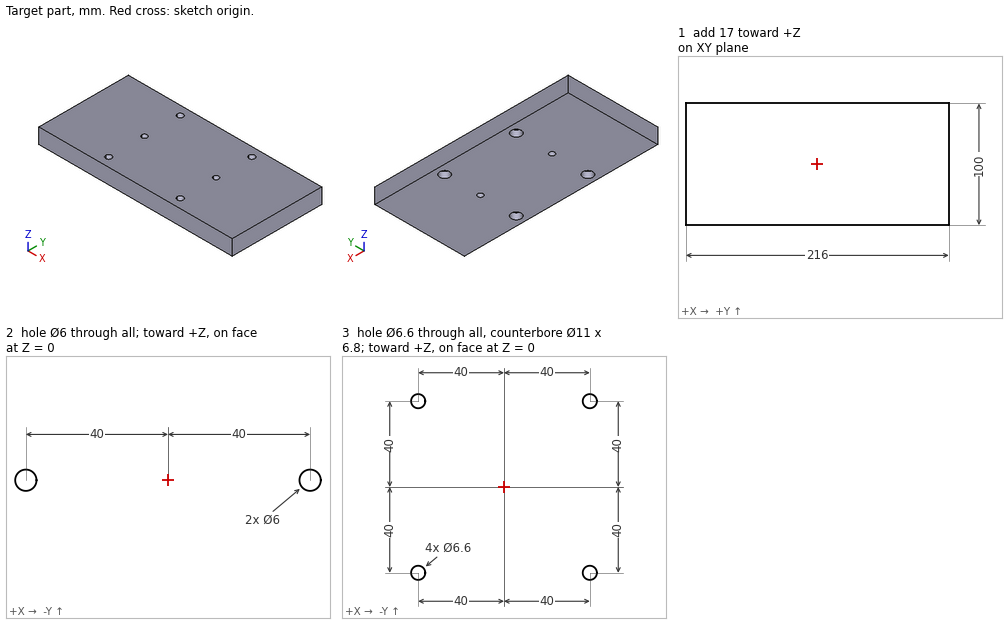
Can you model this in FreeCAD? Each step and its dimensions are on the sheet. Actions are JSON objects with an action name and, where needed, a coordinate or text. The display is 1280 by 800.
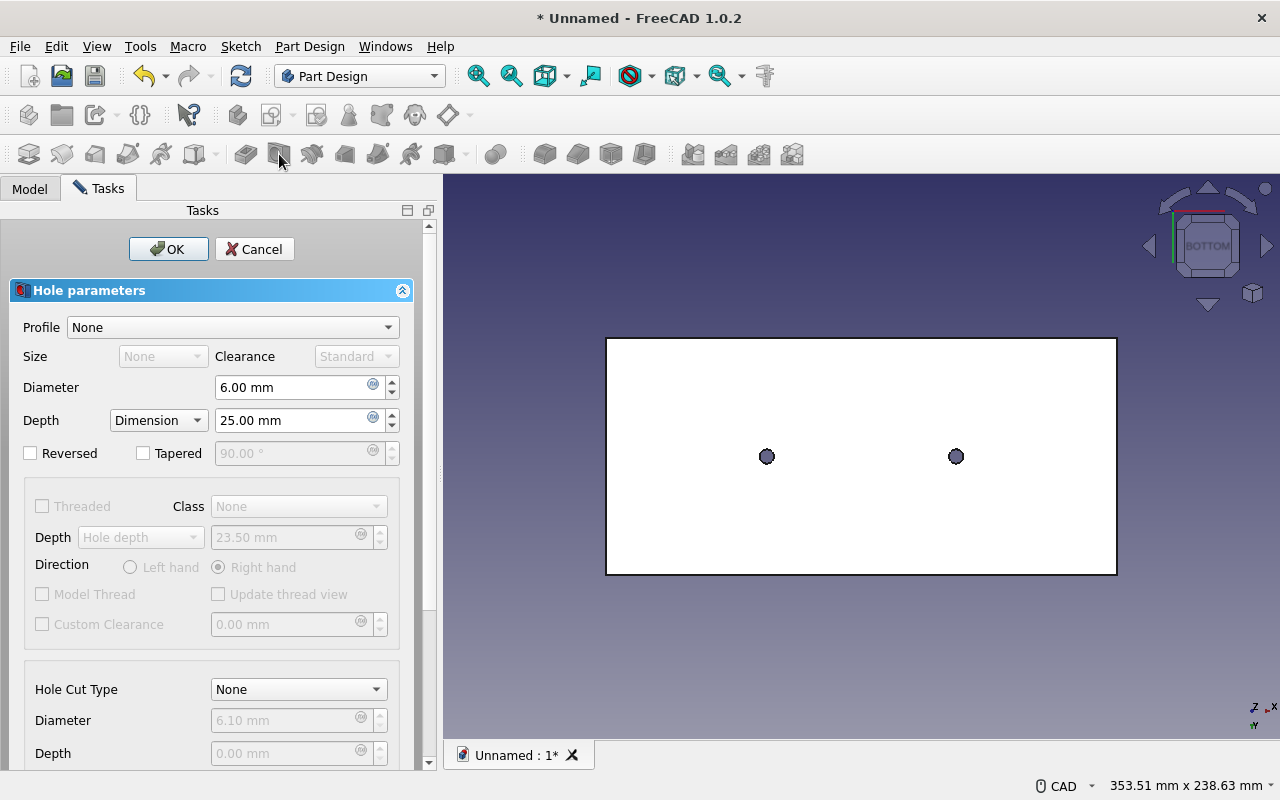
{"action": "triple_click", "coordinate": [300, 388]}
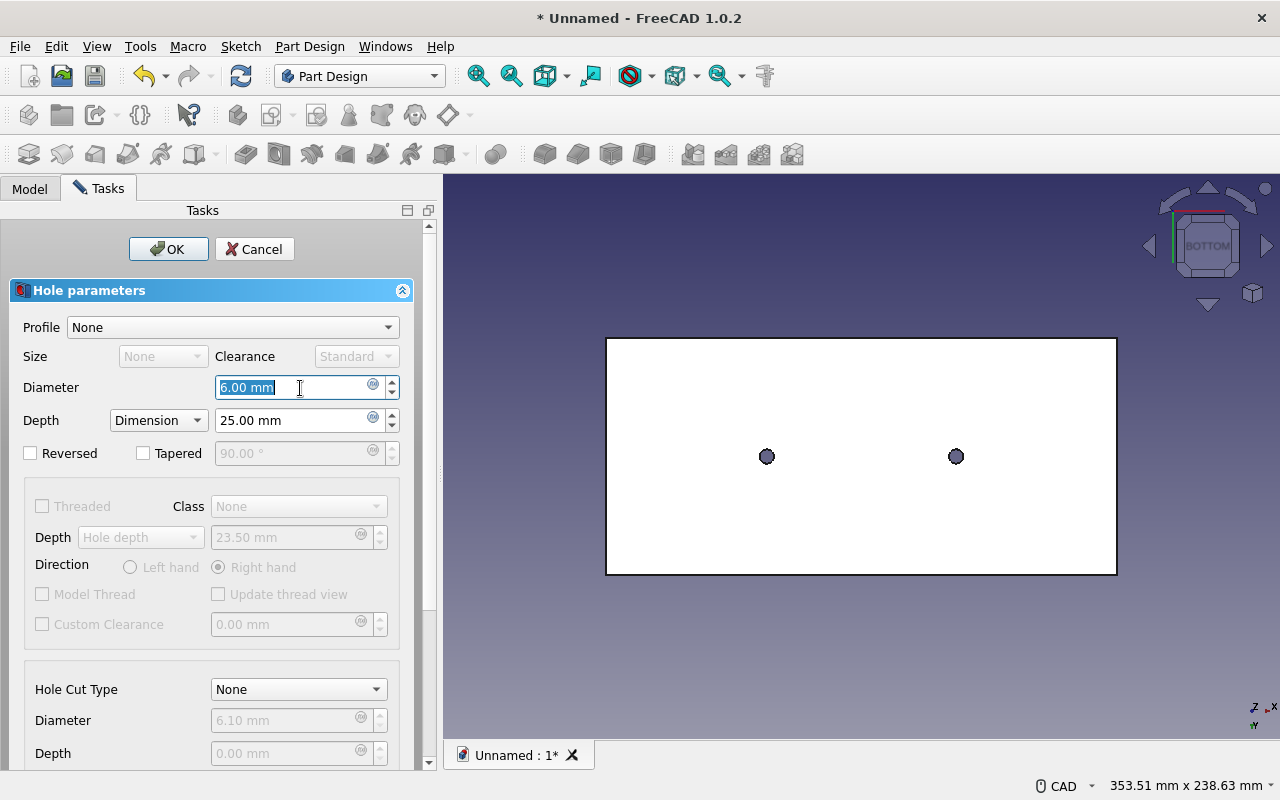
{"action": "type", "text": "6"}
{"action": "key", "text": "Tab"}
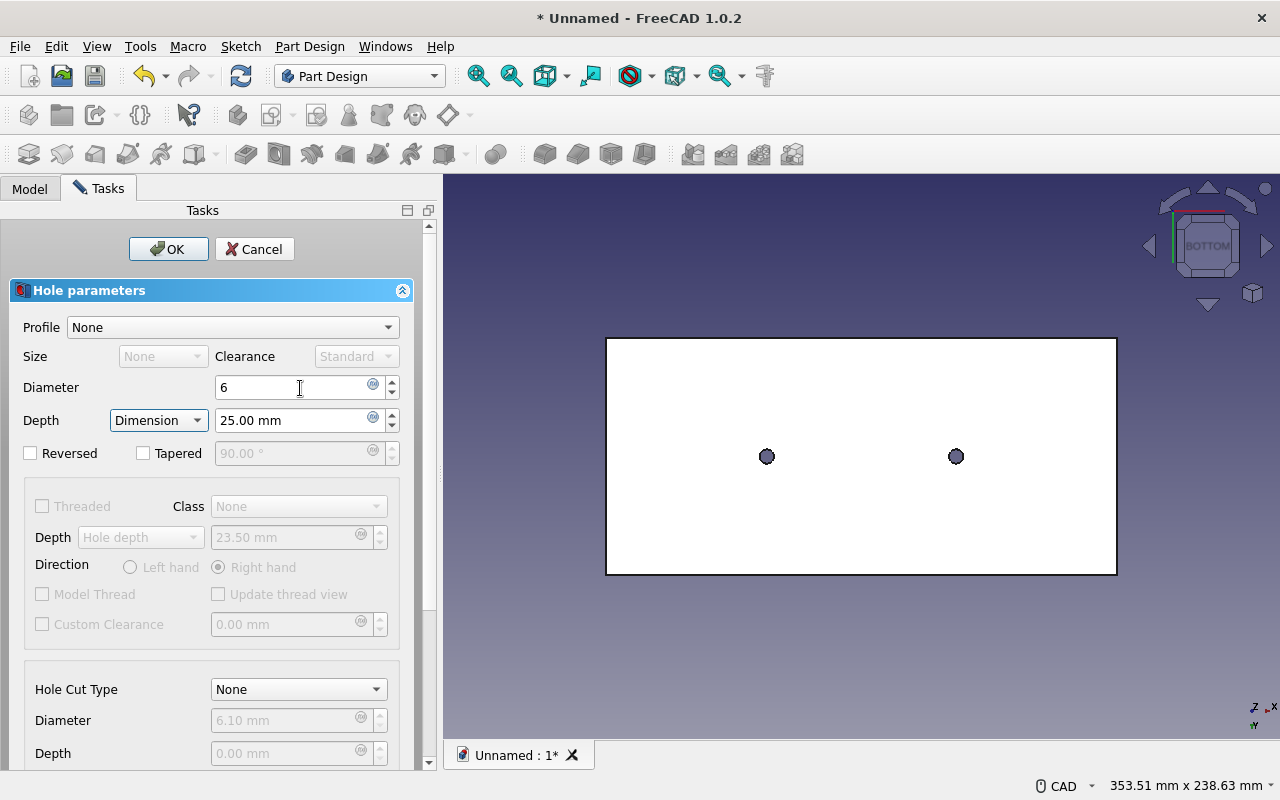
{"action": "left_click", "coordinate": [160, 420]}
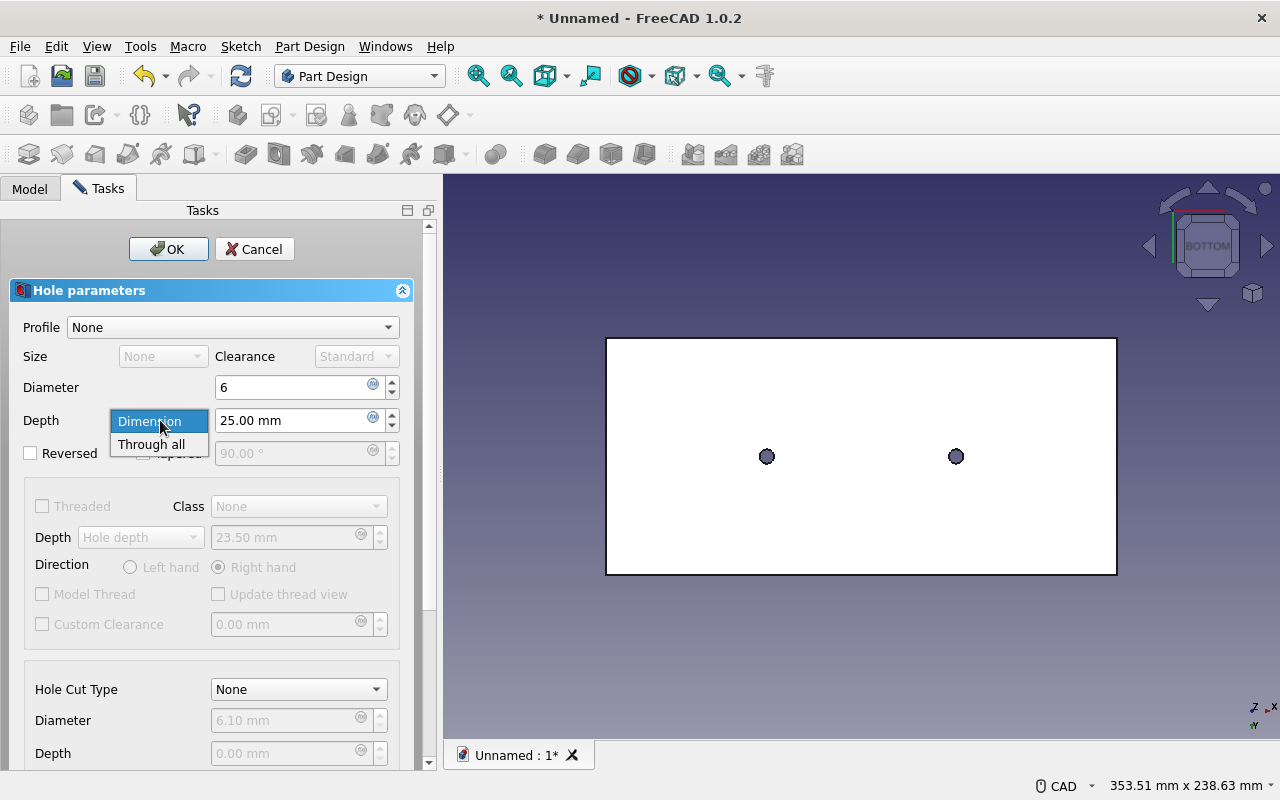
{"action": "left_click", "coordinate": [158, 444]}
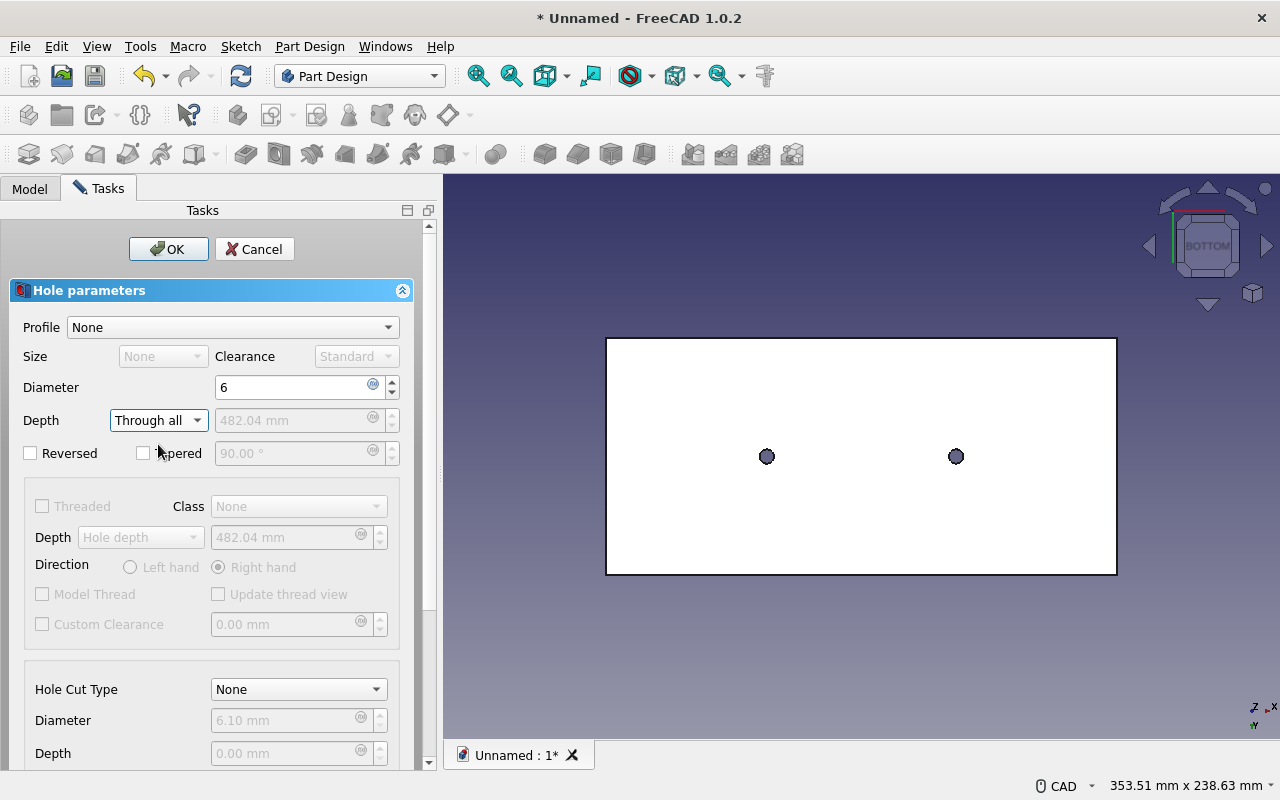
{"action": "left_click", "coordinate": [169, 249]}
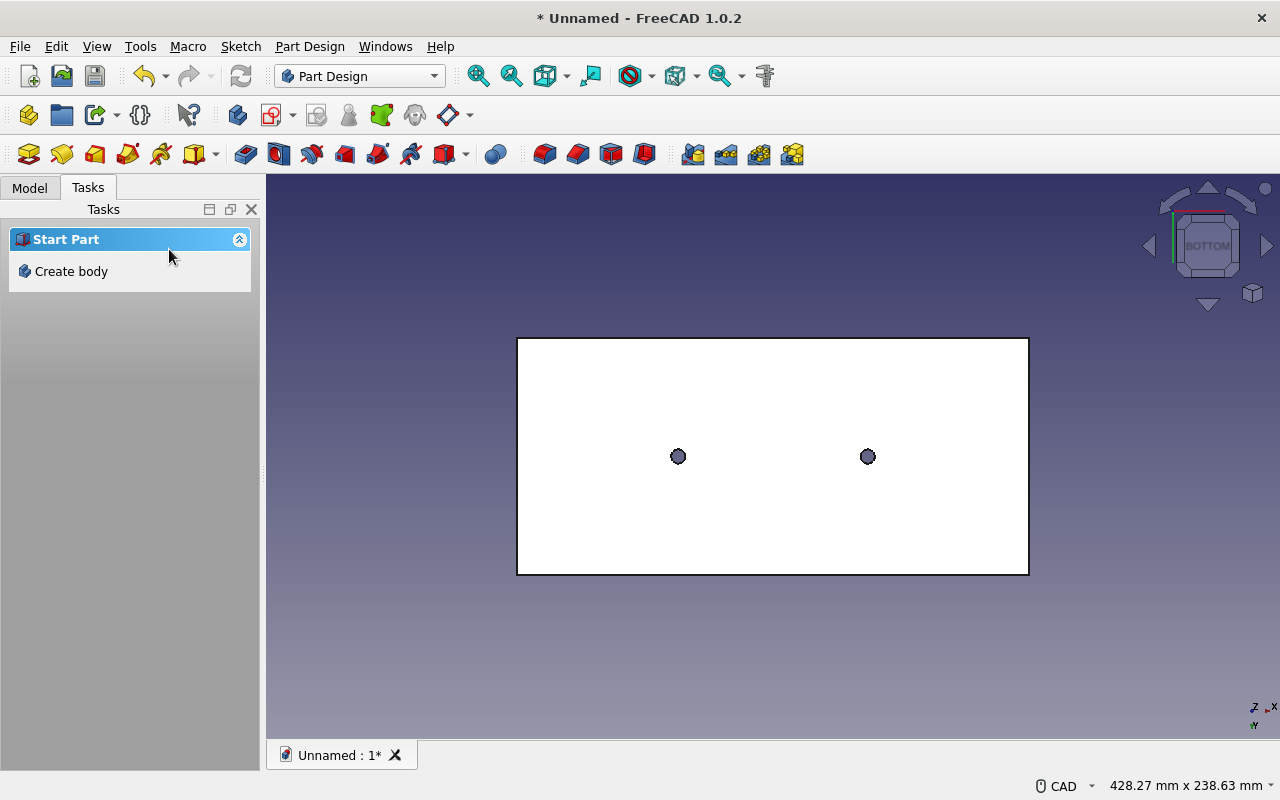
{"action": "left_click", "coordinate": [773, 456]}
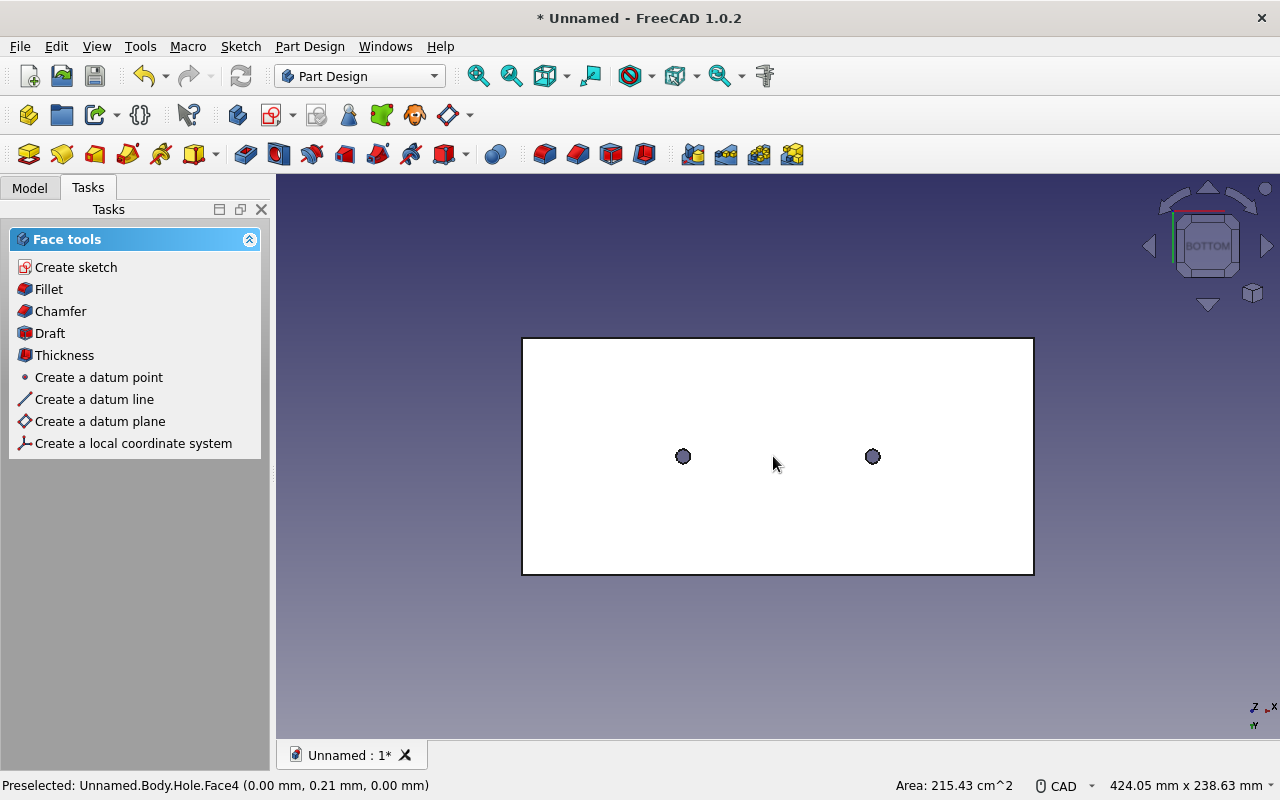
{"action": "left_click", "coordinate": [270, 116]}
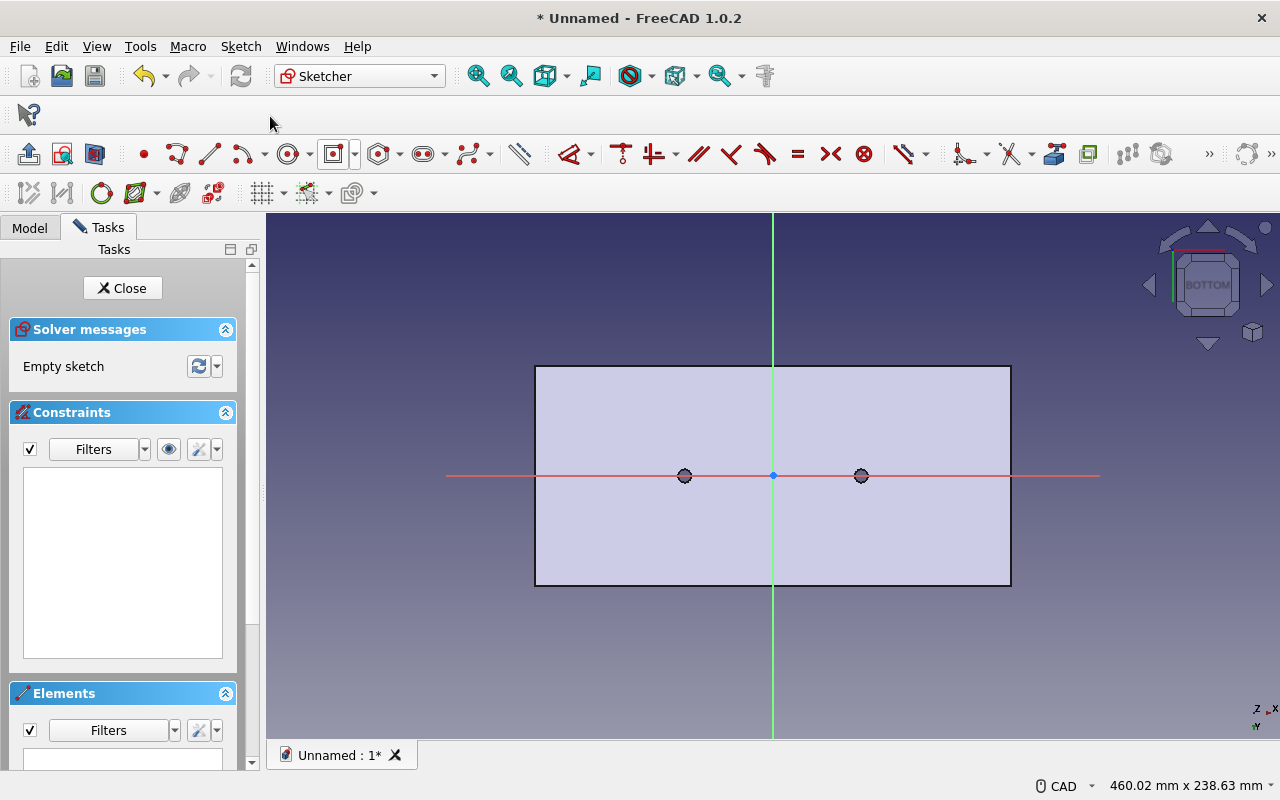
{"action": "scroll", "coordinate": [856, 476], "scroll_direction": "up", "scroll_amount": 3}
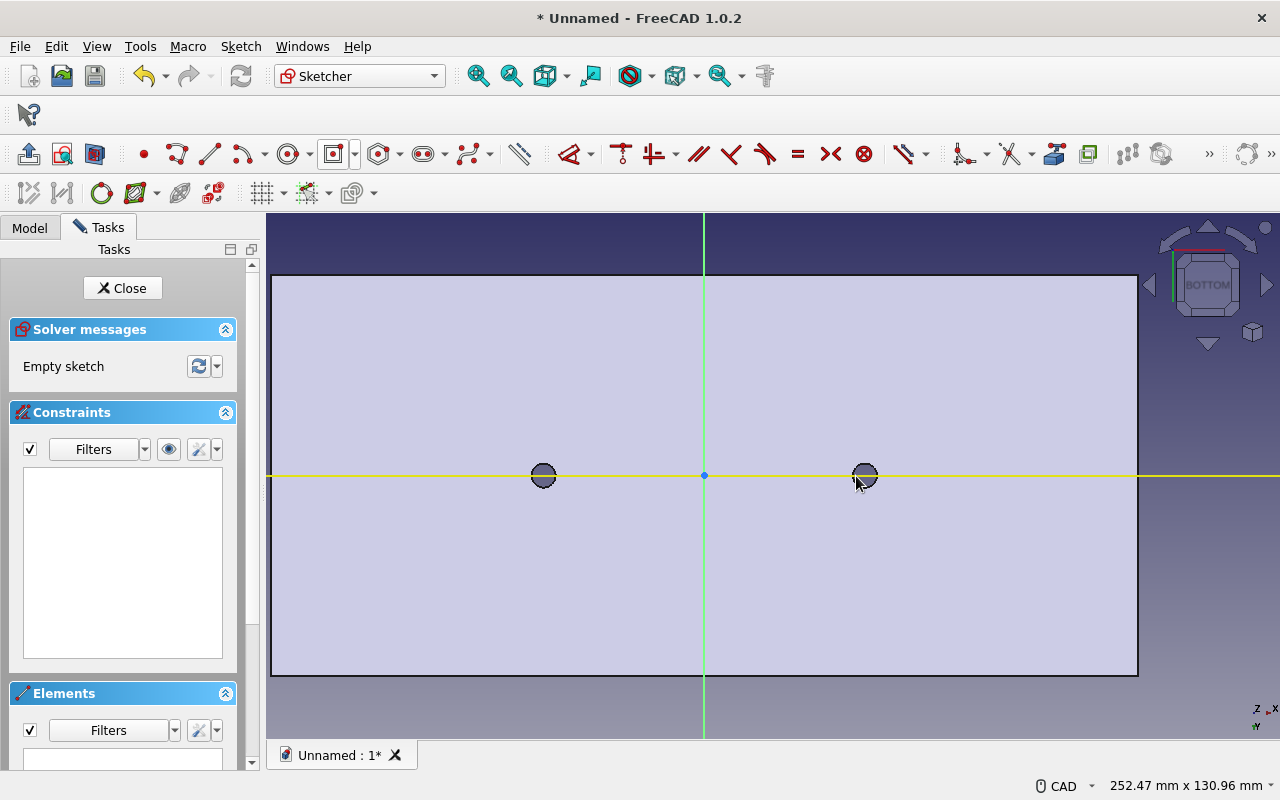
{"action": "left_click", "coordinate": [288, 154]}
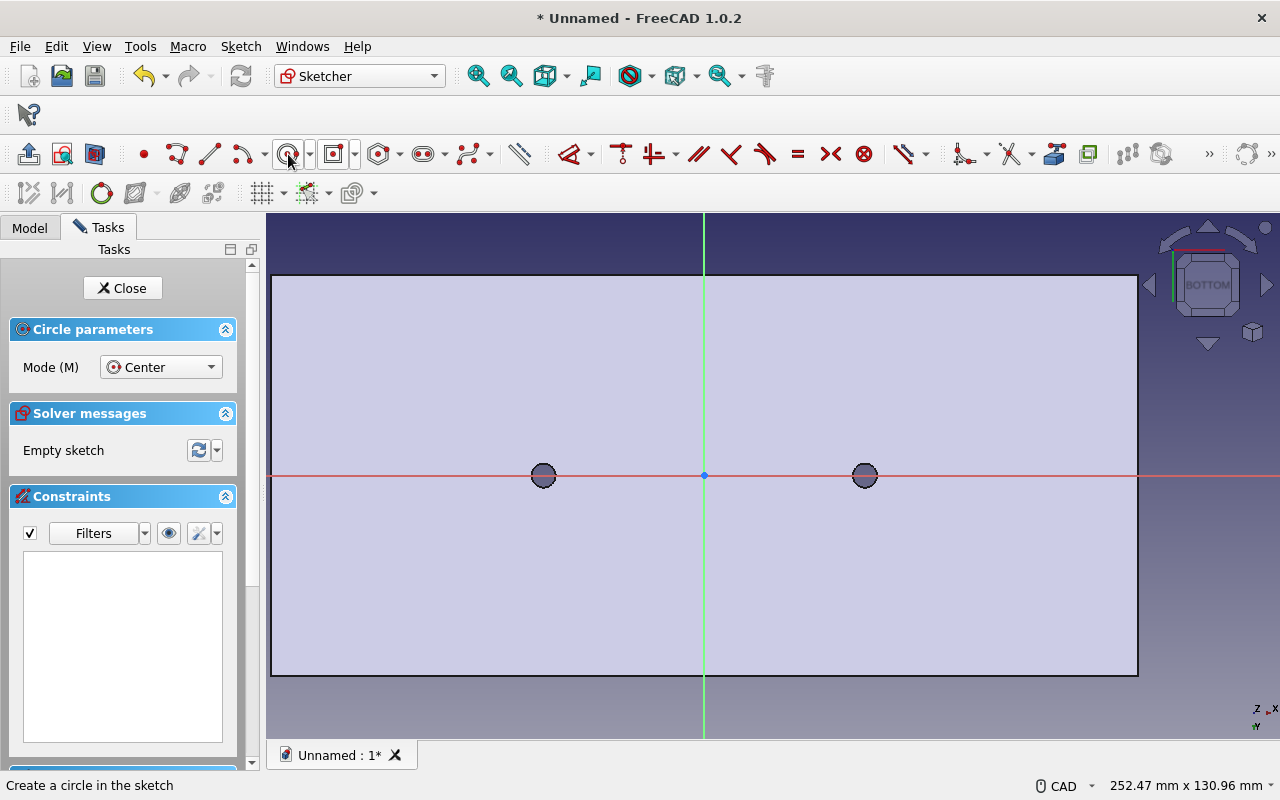
{"action": "scroll", "coordinate": [544, 636], "scroll_direction": "up", "scroll_amount": 3}